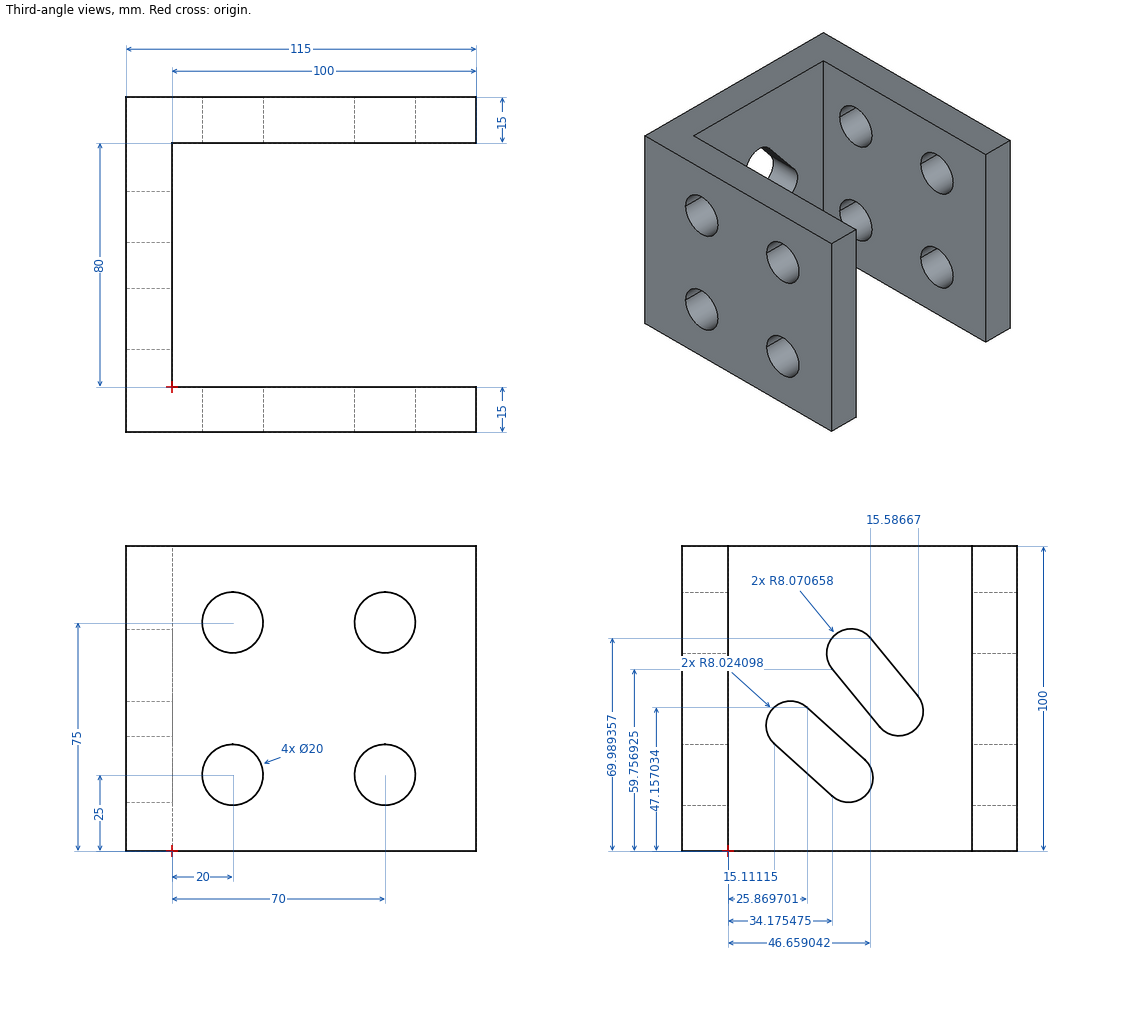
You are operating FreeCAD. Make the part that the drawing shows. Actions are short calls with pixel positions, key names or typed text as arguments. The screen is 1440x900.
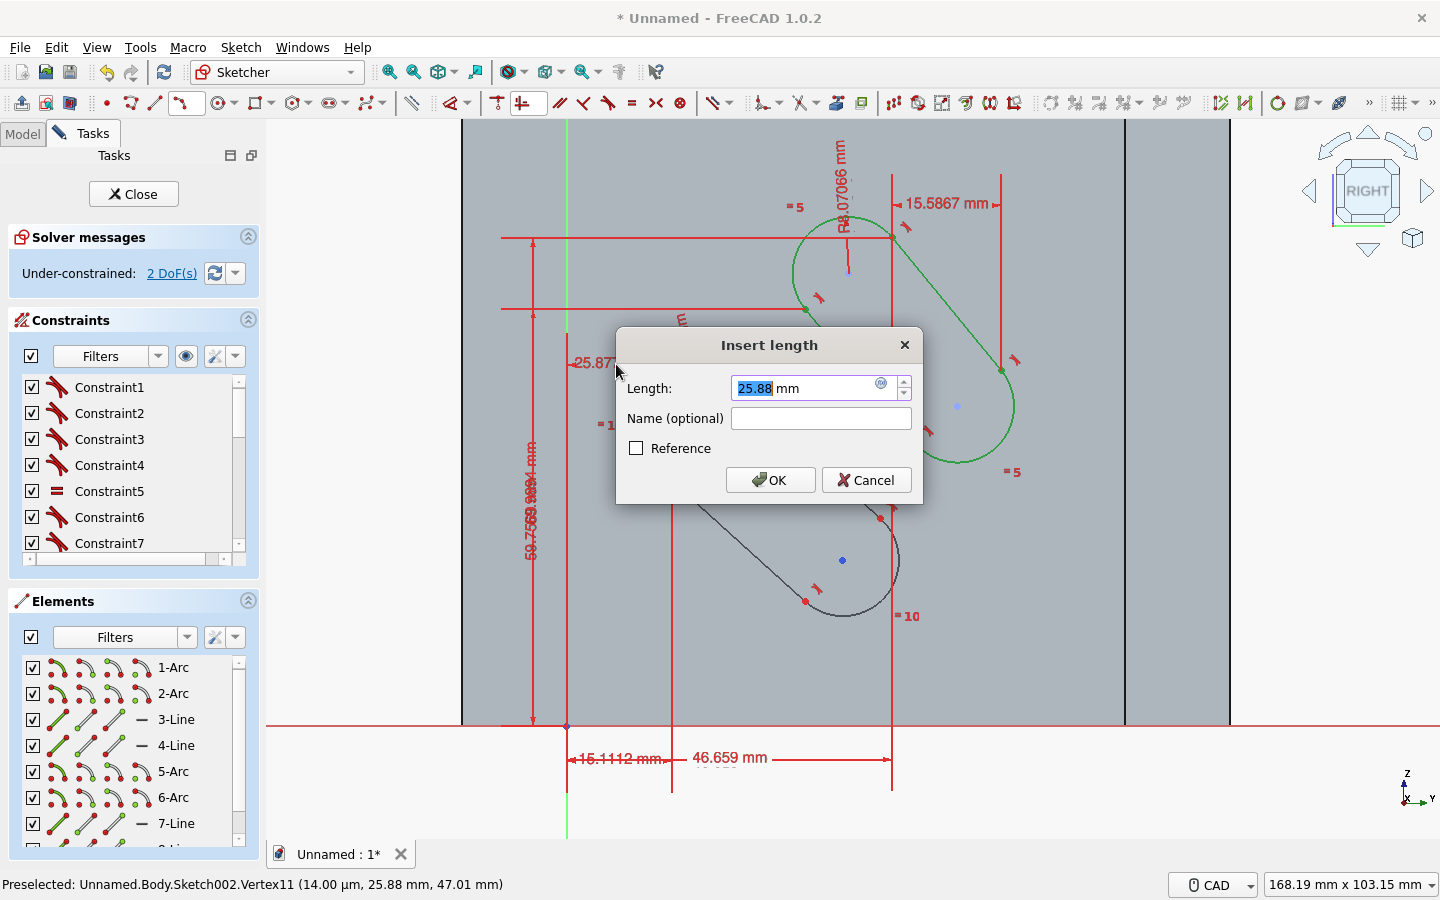
text(25.869701)
key(Return)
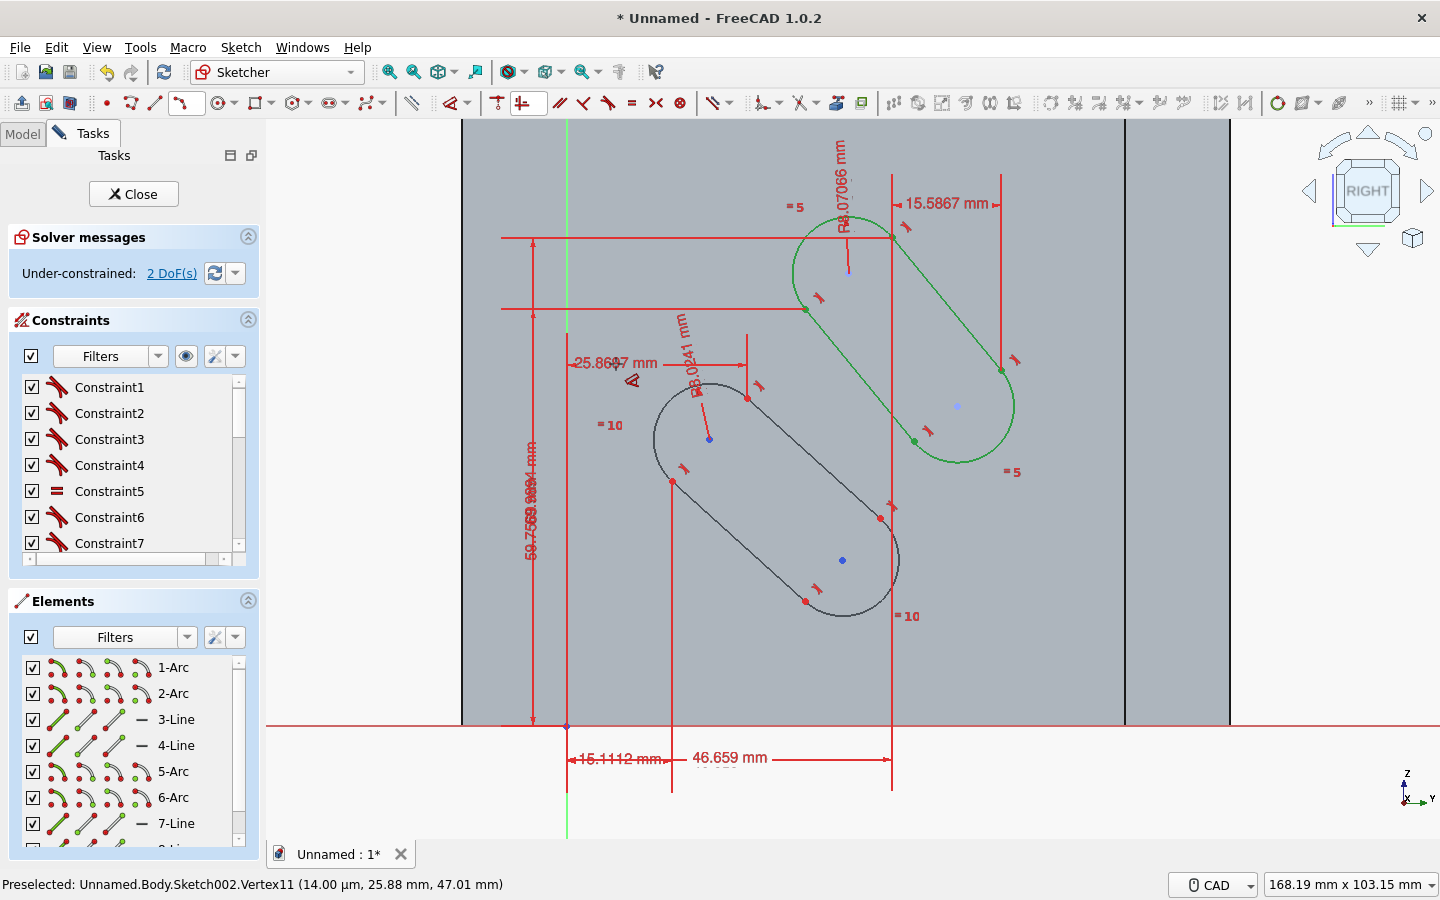
click(747, 398)
click(533, 562)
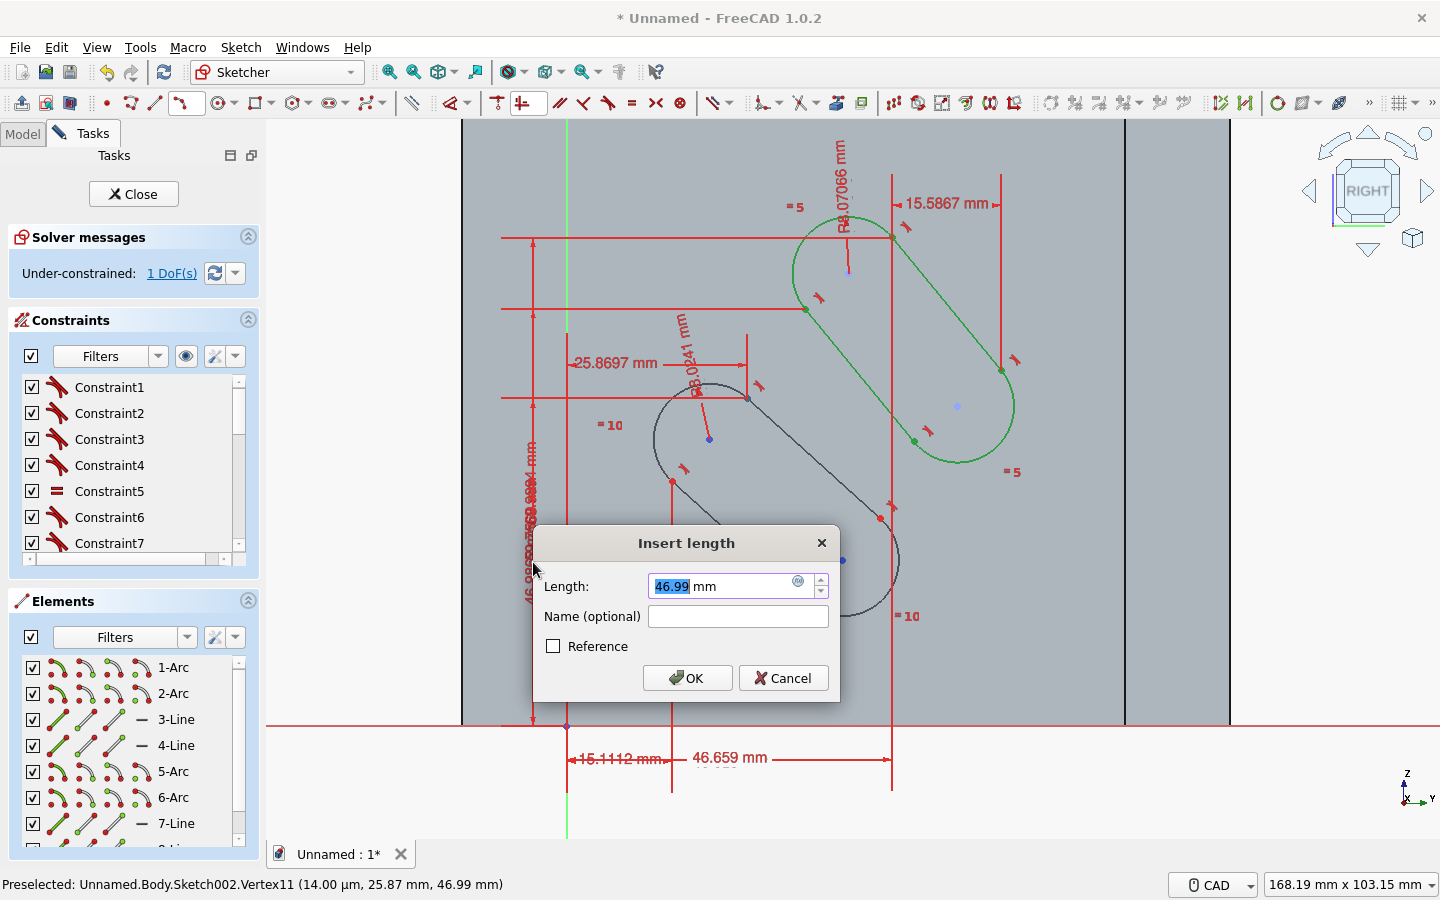
text(47.157034)
key(Return)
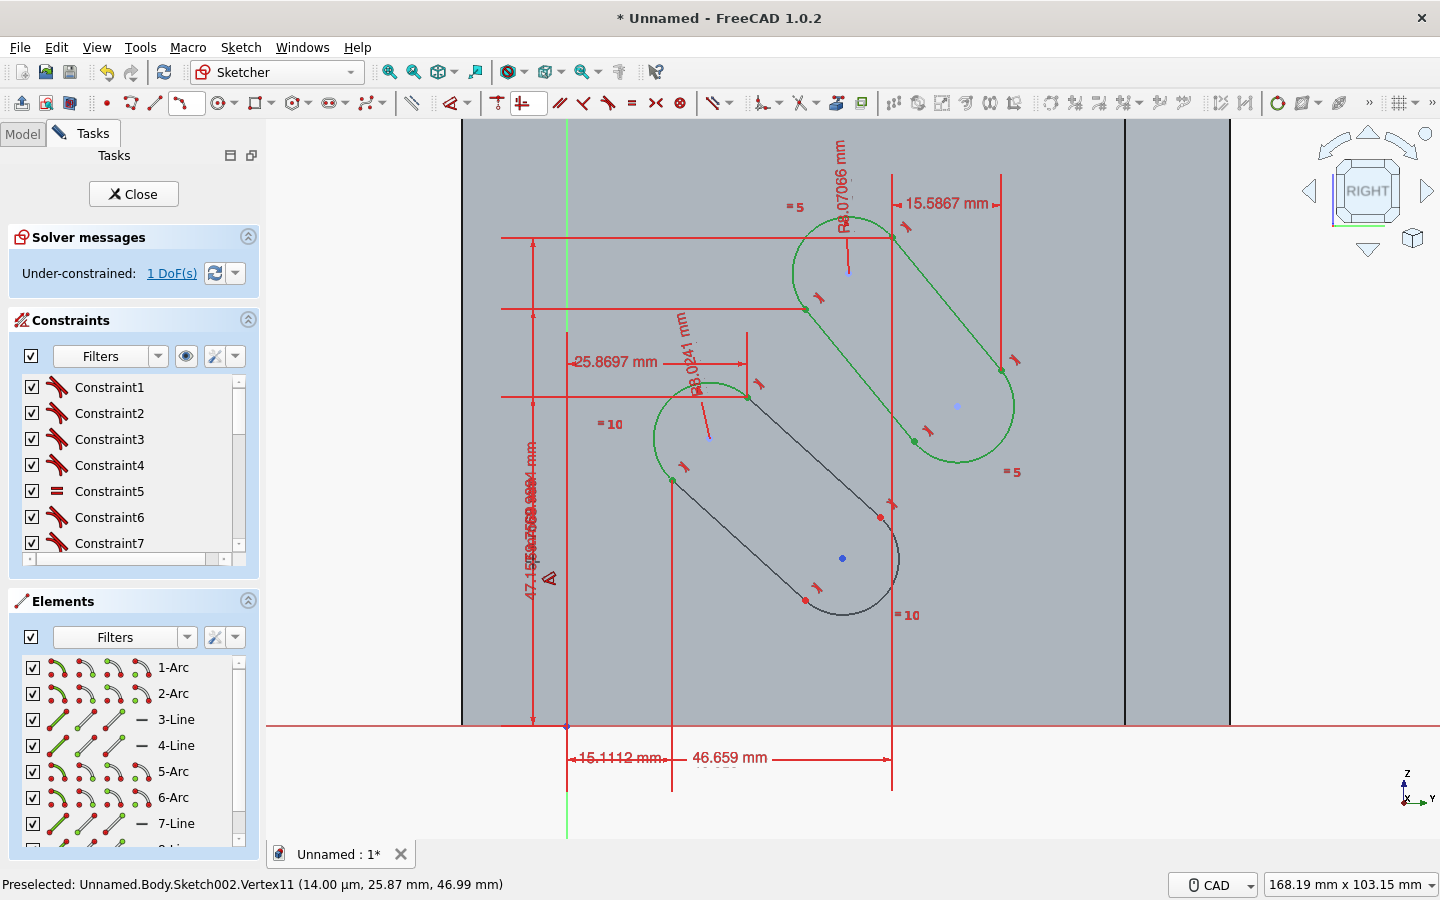
click(805, 600)
click(686, 566)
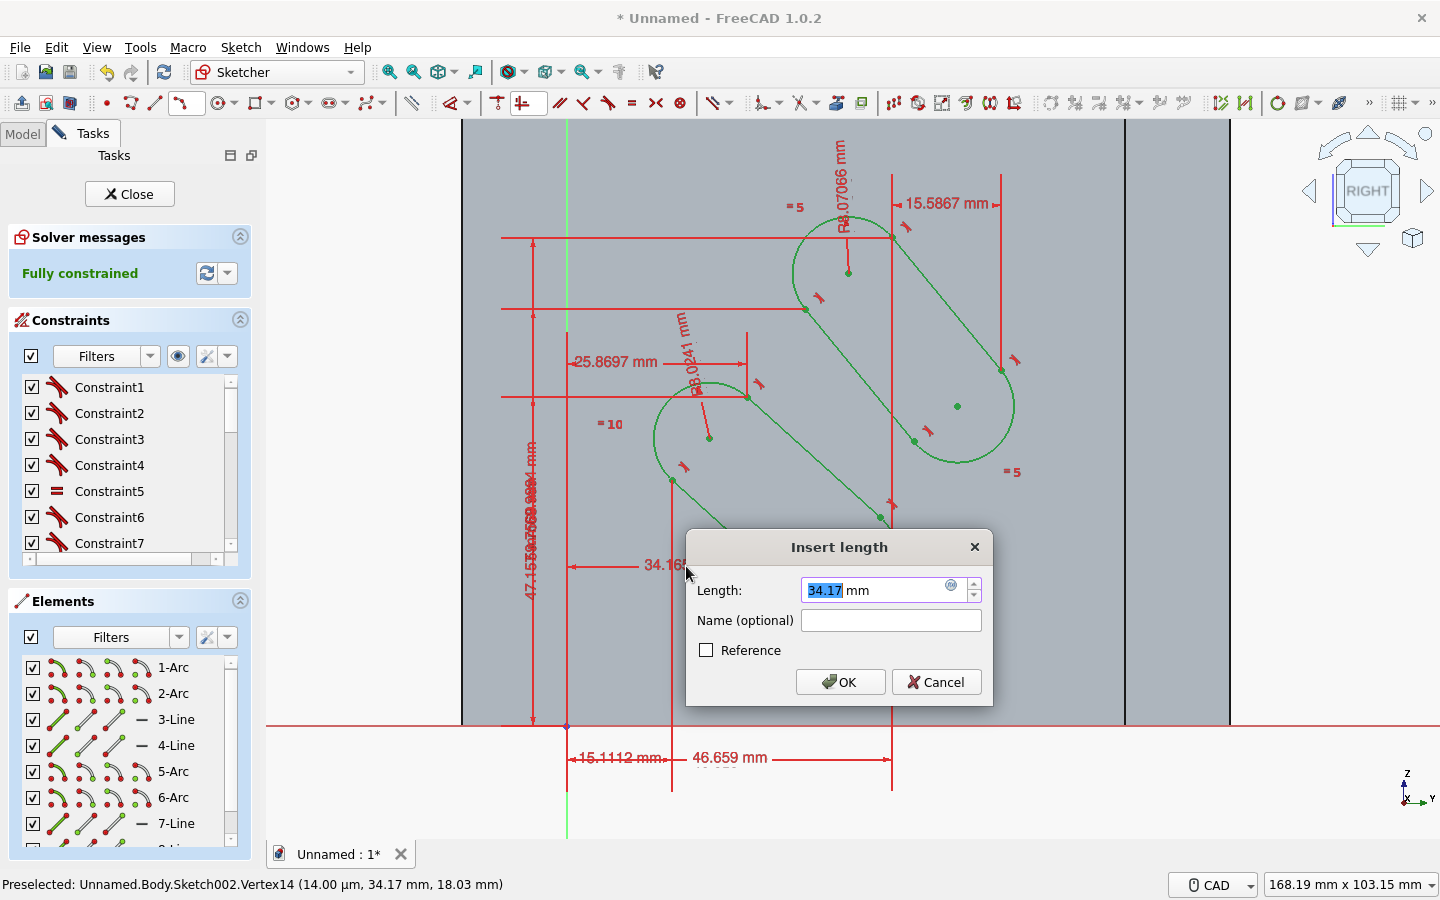
text(34.175475)
key(Return)
key(Escape)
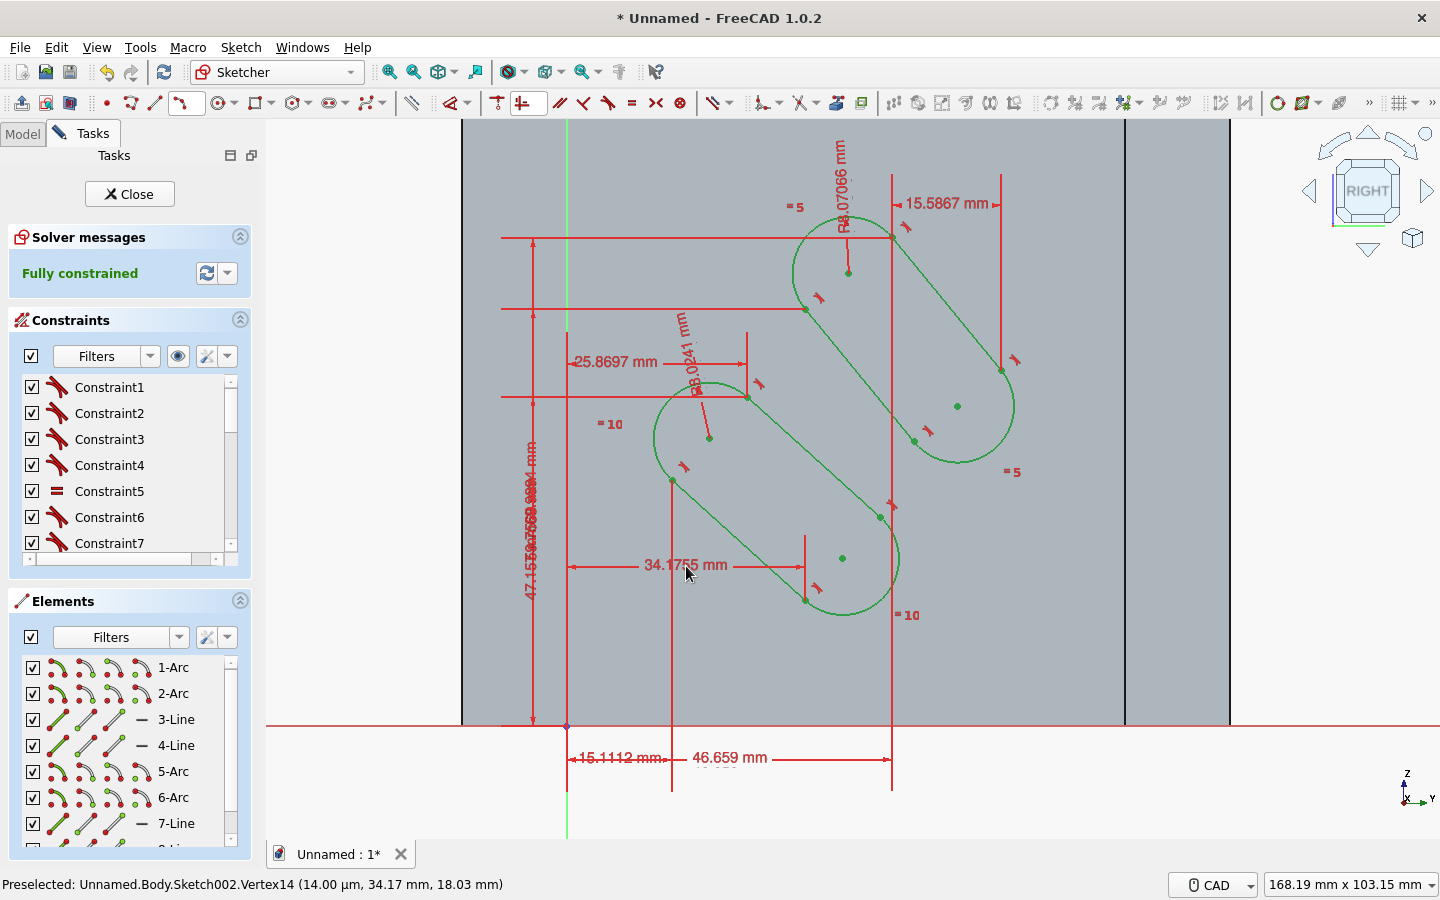
click(130, 194)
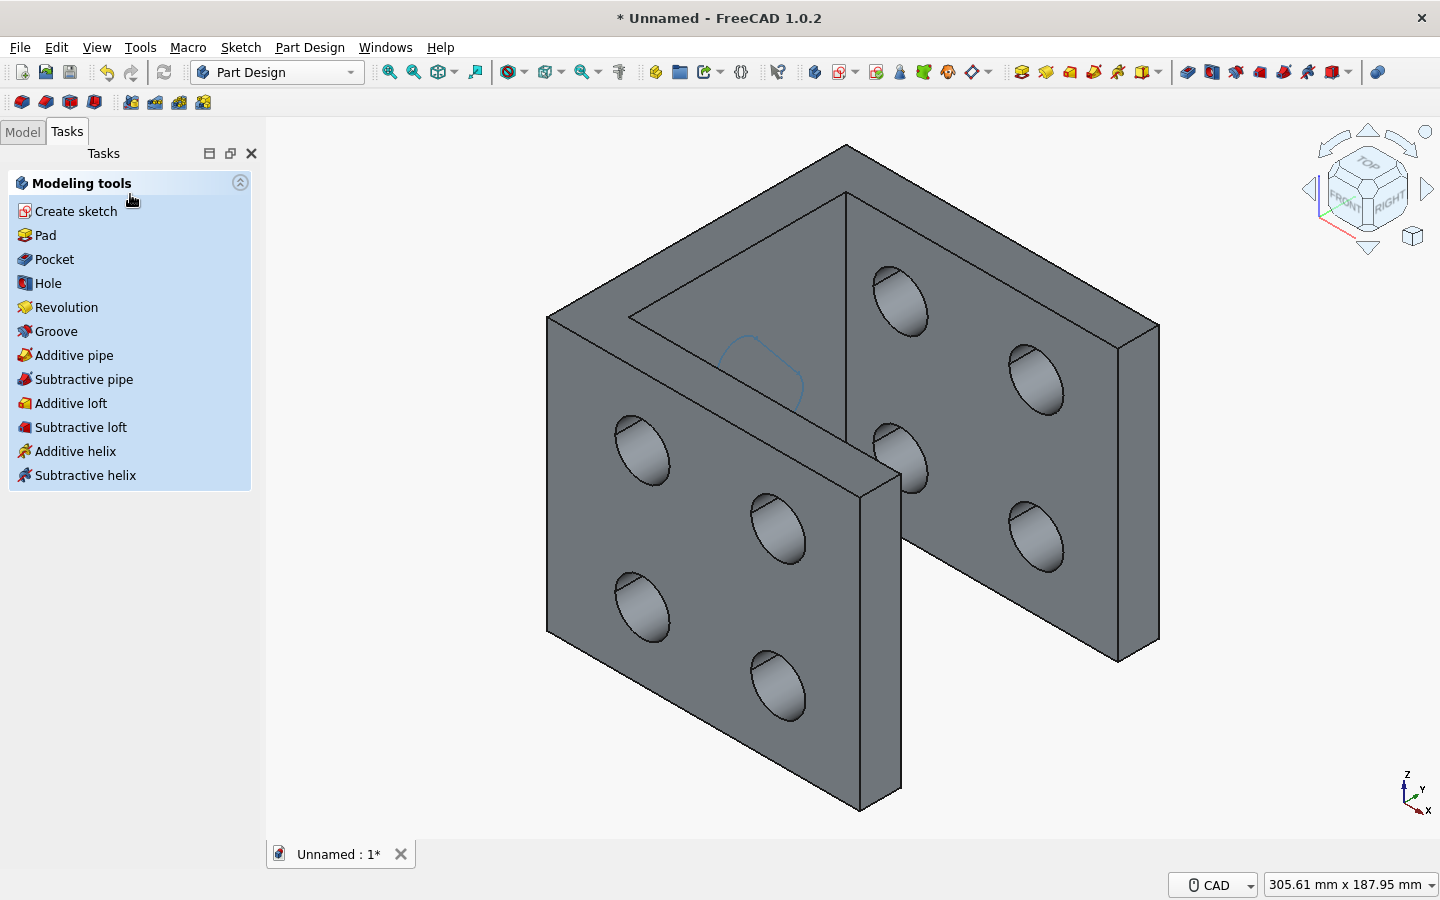
click(1188, 72)